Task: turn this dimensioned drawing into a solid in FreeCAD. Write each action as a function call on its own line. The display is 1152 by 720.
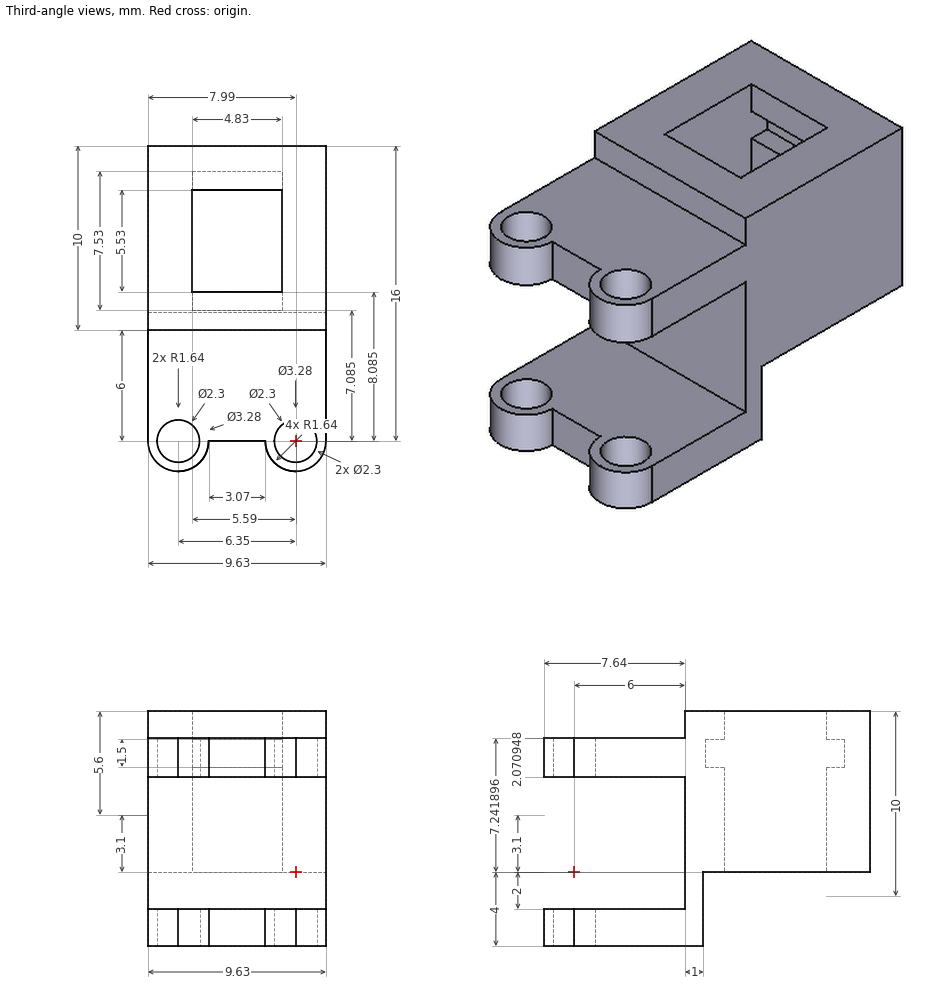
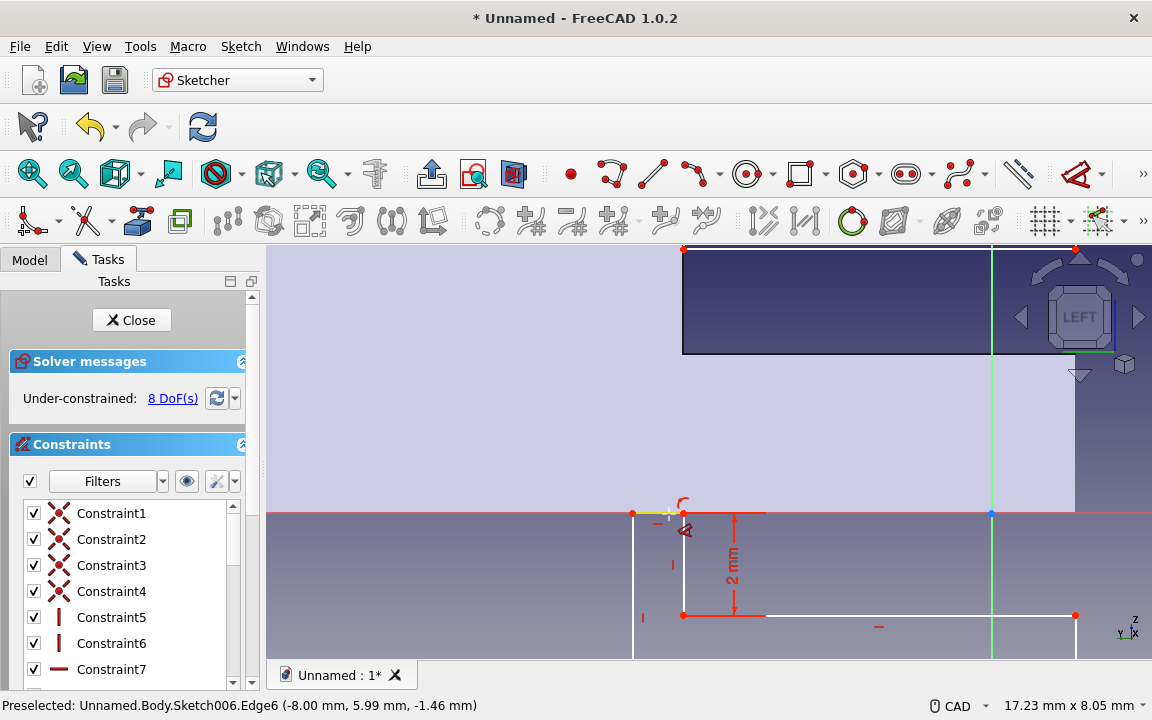
click(669, 513)
click(658, 547)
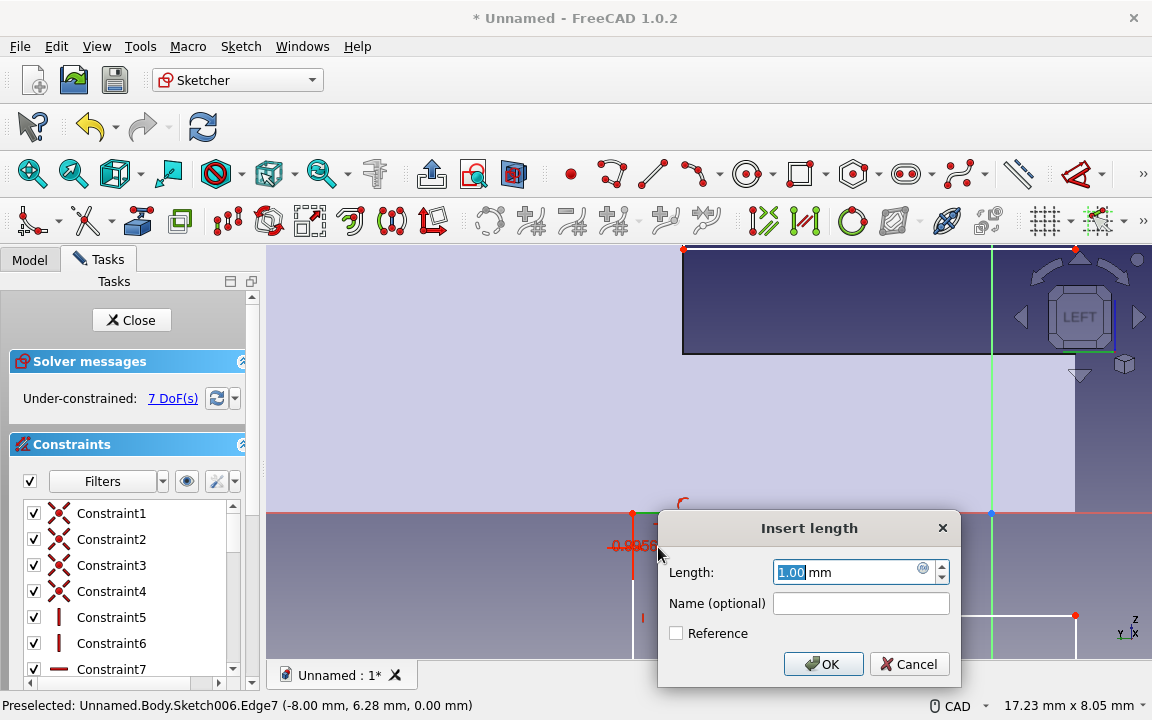
text(1)
key(Return)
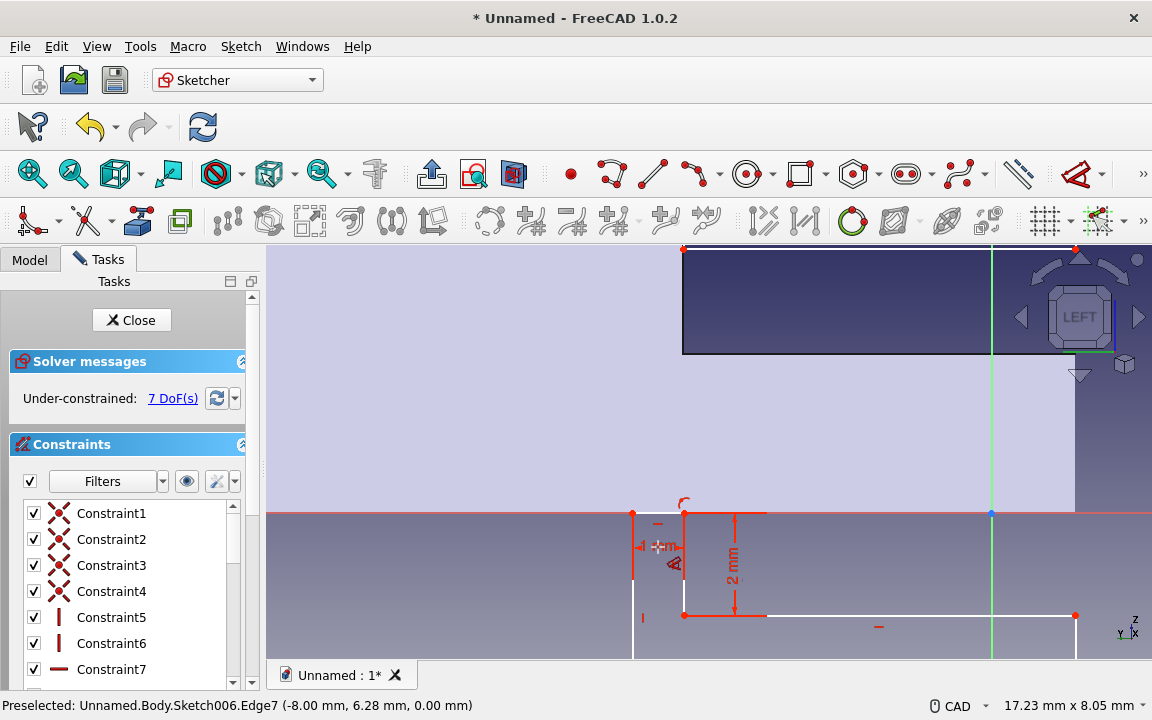
click(633, 575)
click(599, 572)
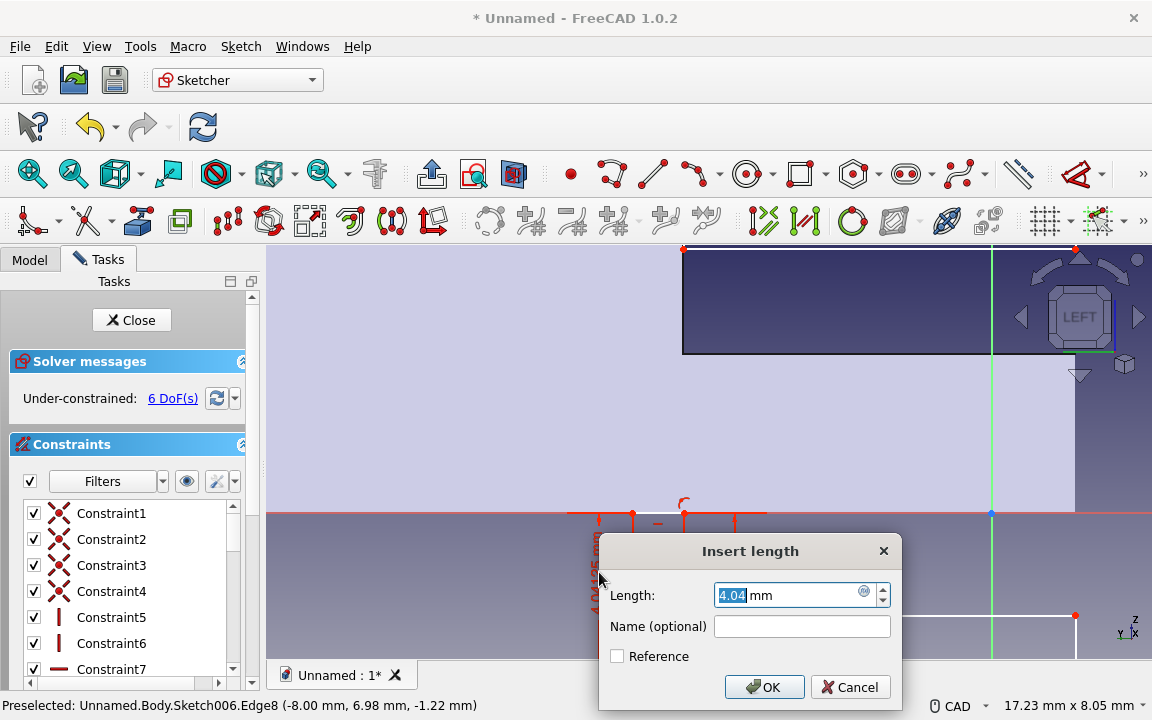
text(4)
key(Return)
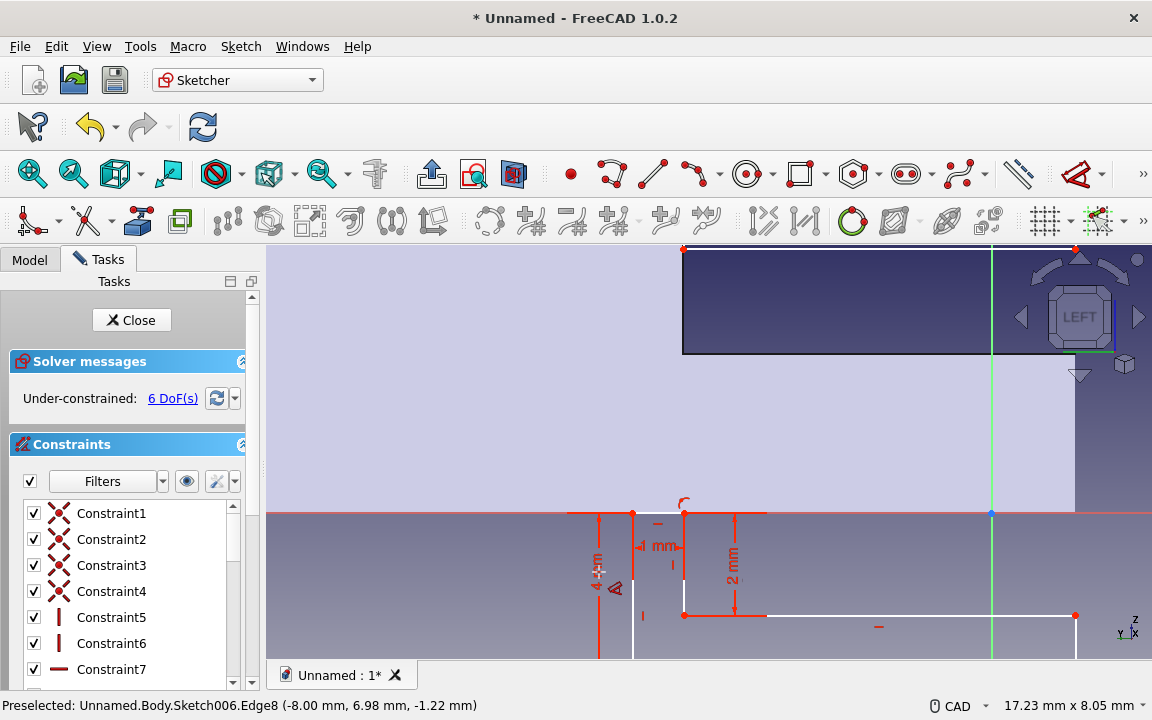
scroll(466, 470, down, 4)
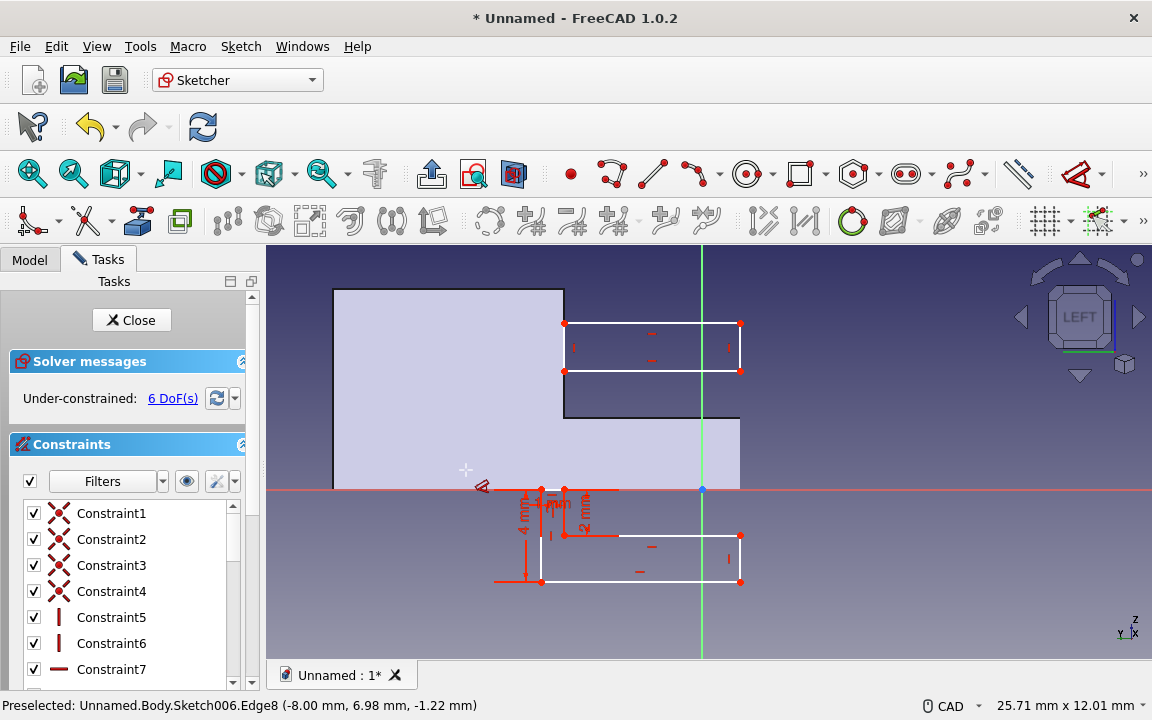
click(564, 323)
click(633, 289)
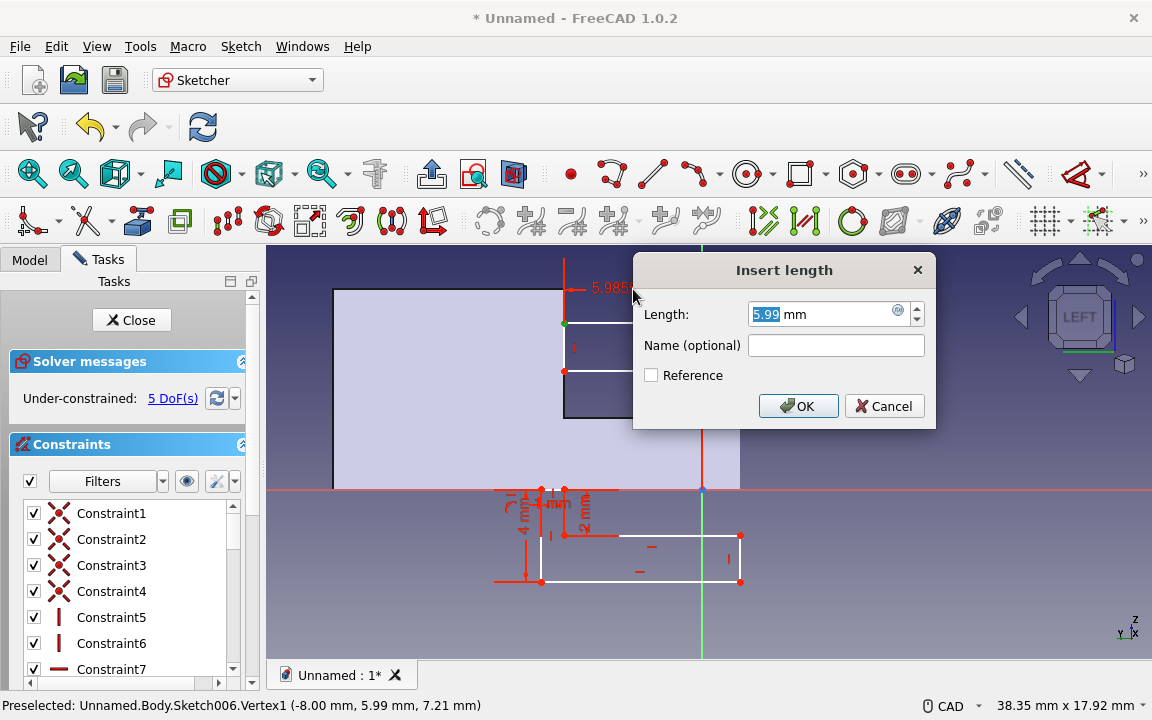
text(6)
key(Return)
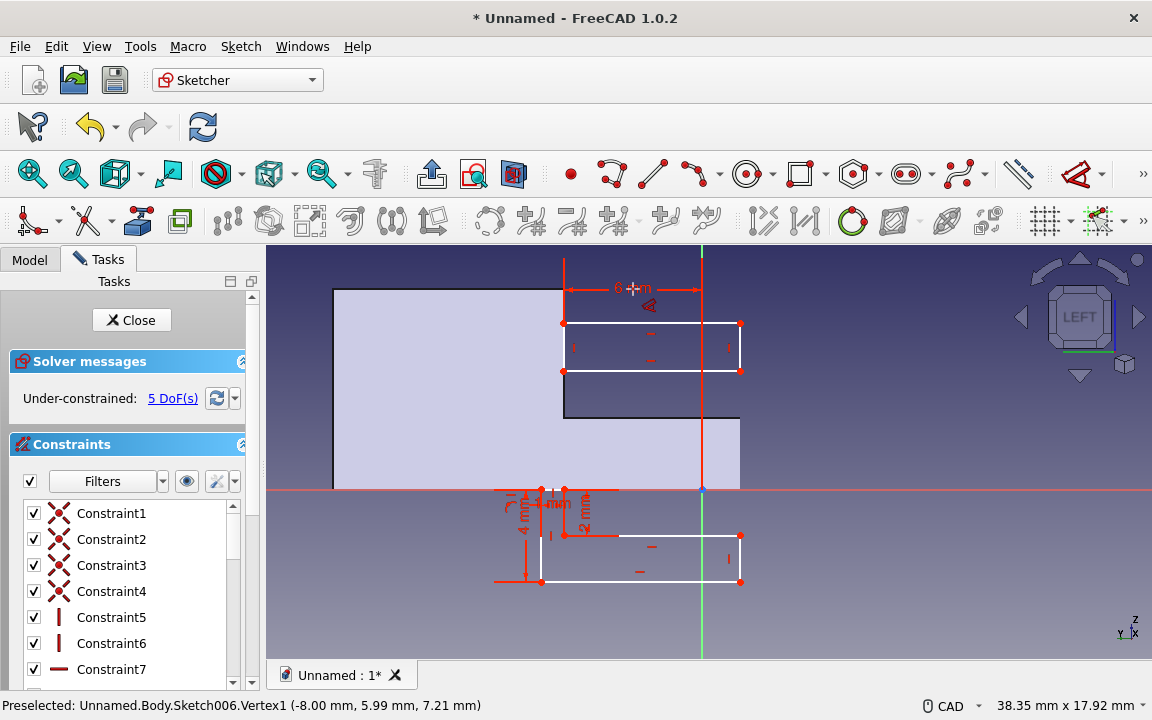
click(564, 536)
click(633, 456)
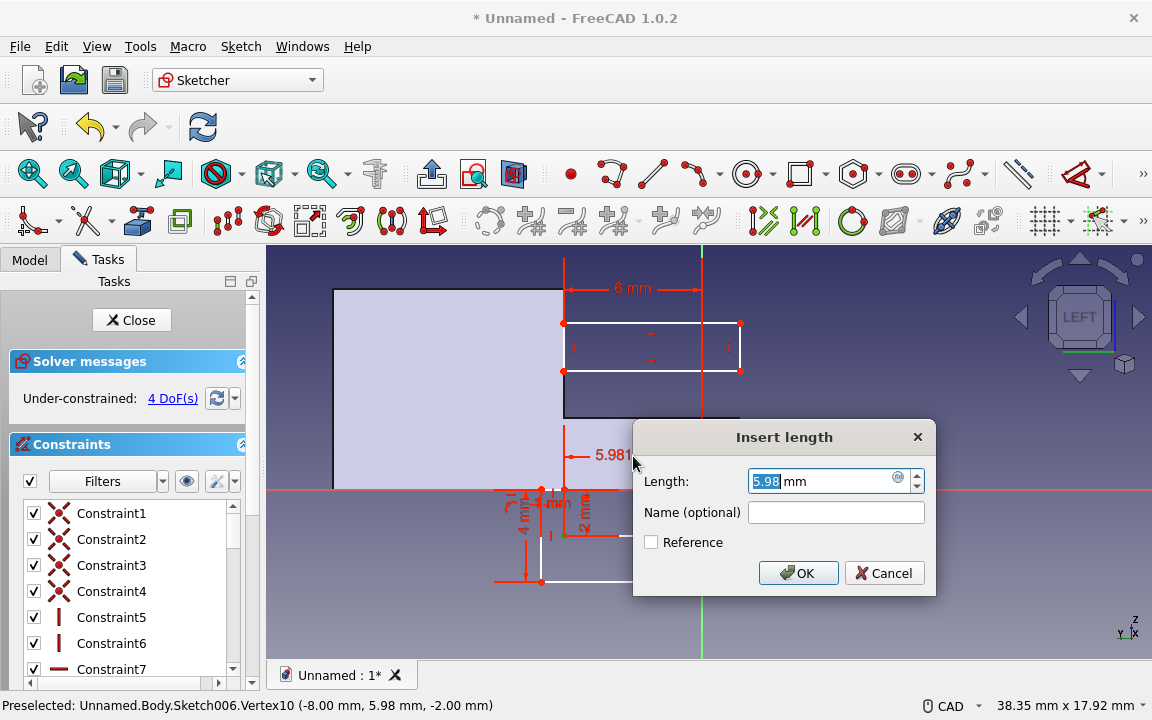
text(6)
key(Return)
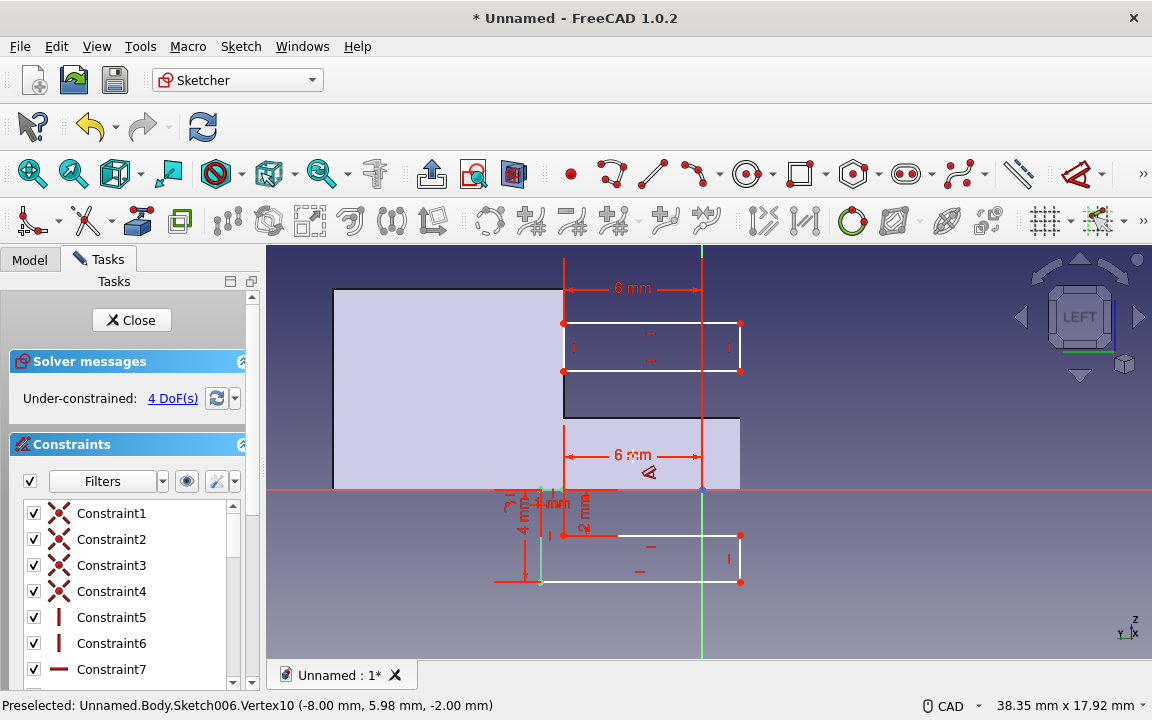
click(617, 371)
click(652, 337)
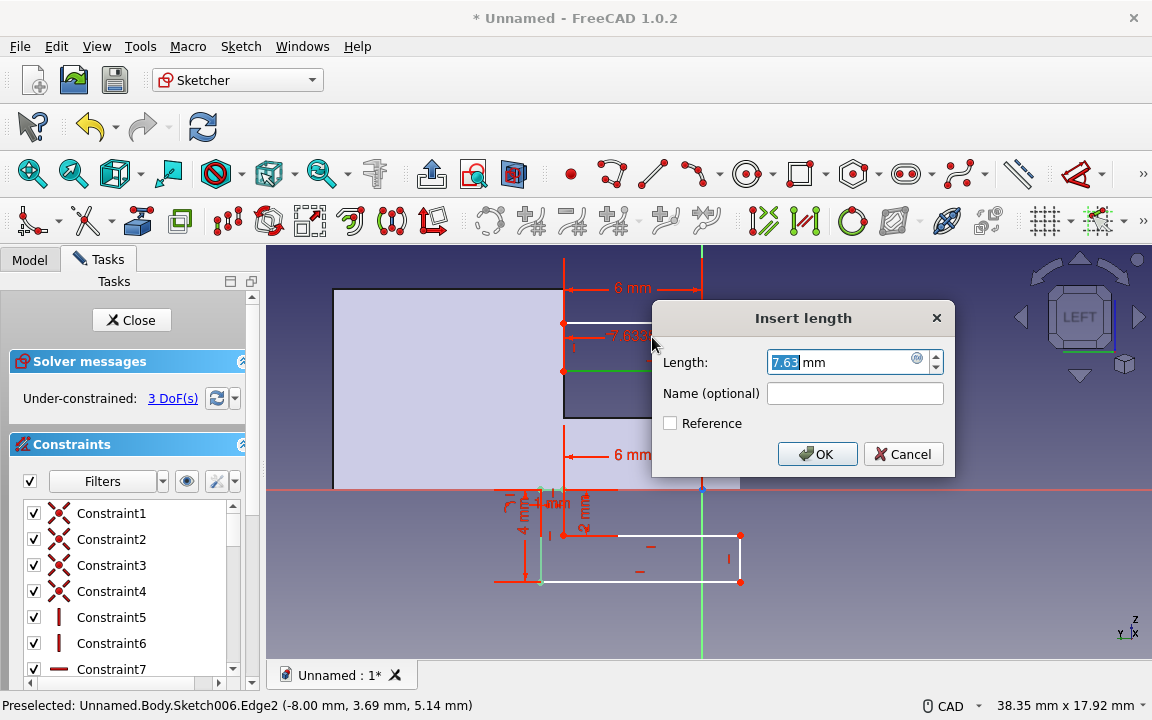
text(7.64)
key(Return)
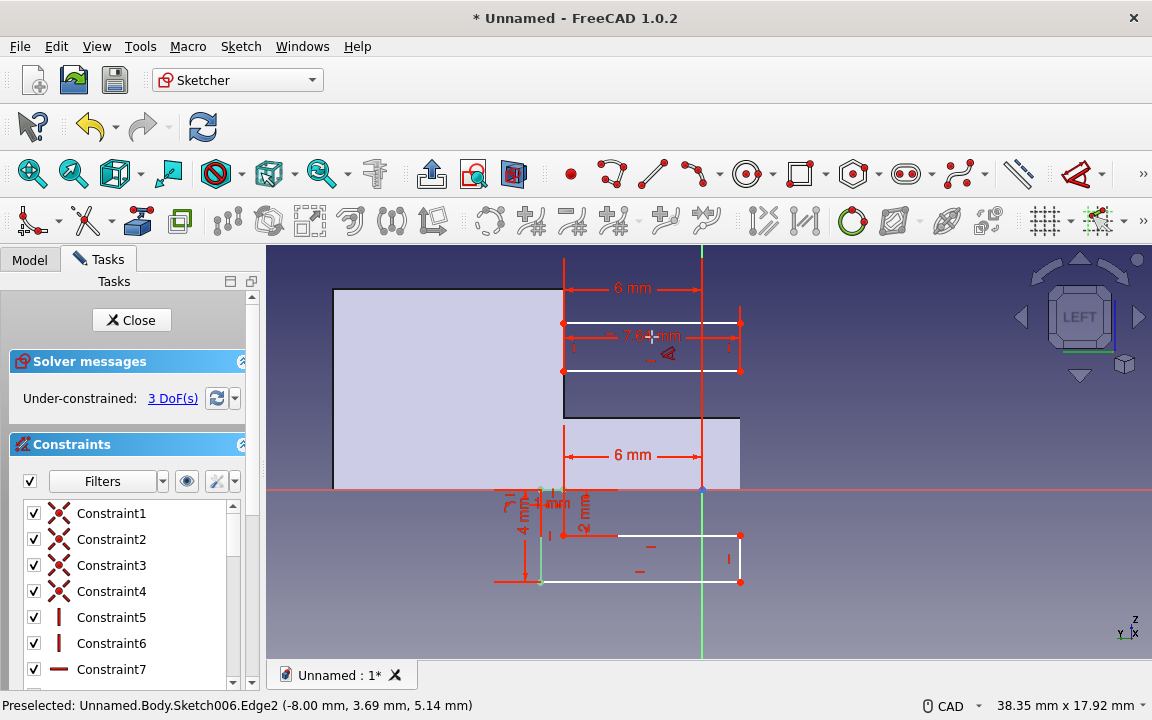
click(687, 536)
click(652, 618)